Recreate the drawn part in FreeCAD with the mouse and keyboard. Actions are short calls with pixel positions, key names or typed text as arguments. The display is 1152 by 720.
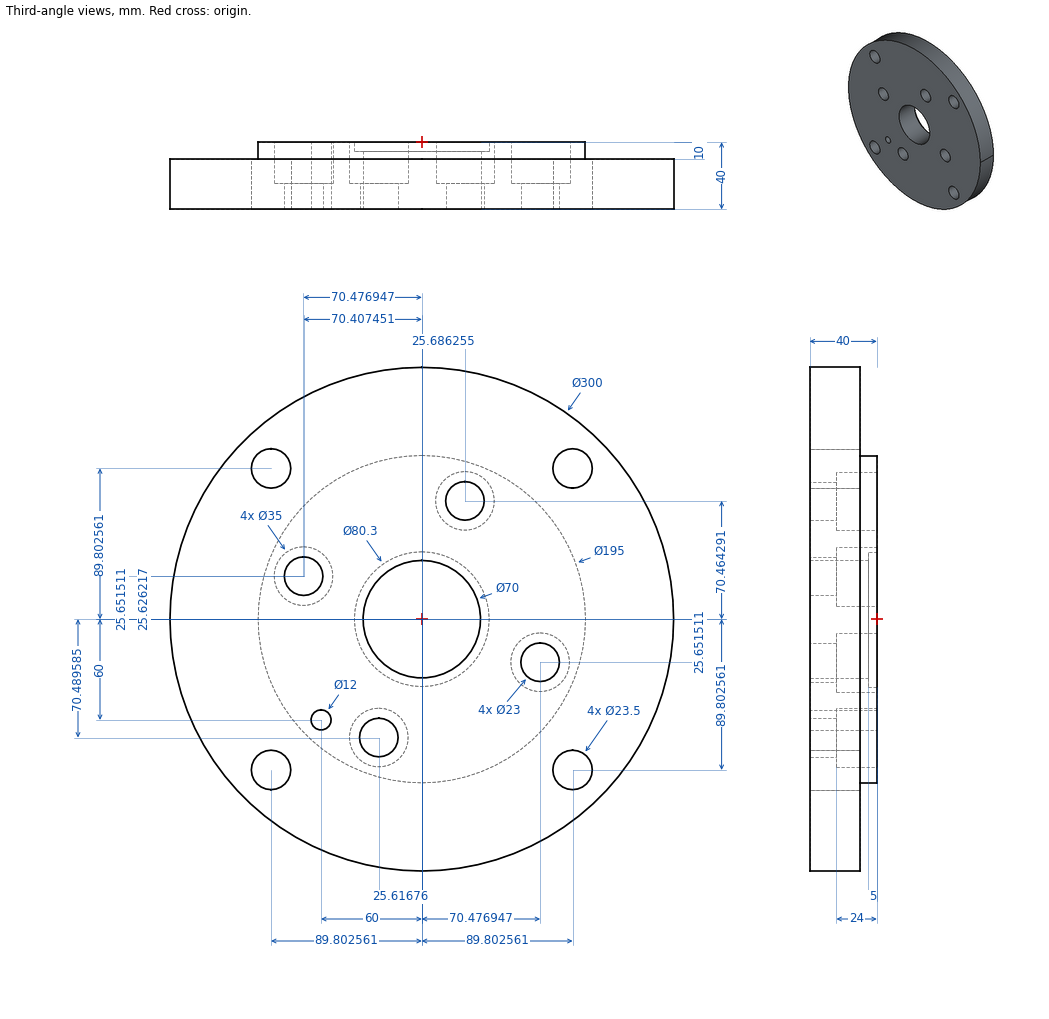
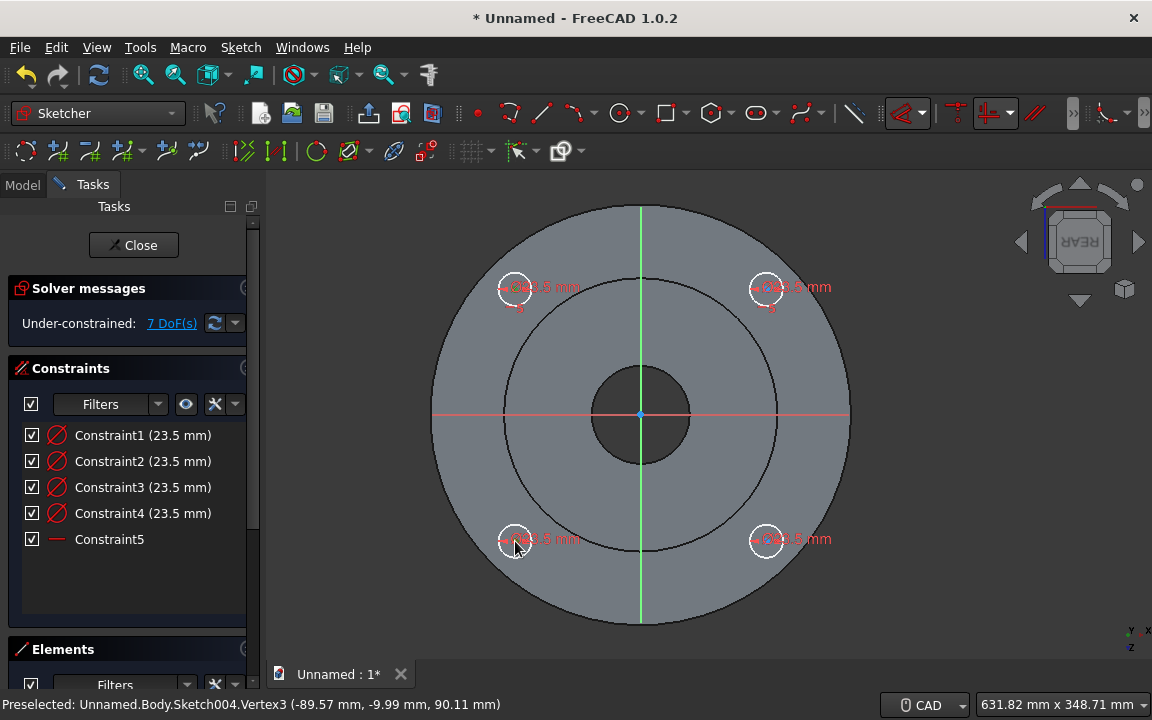
click(1012, 114)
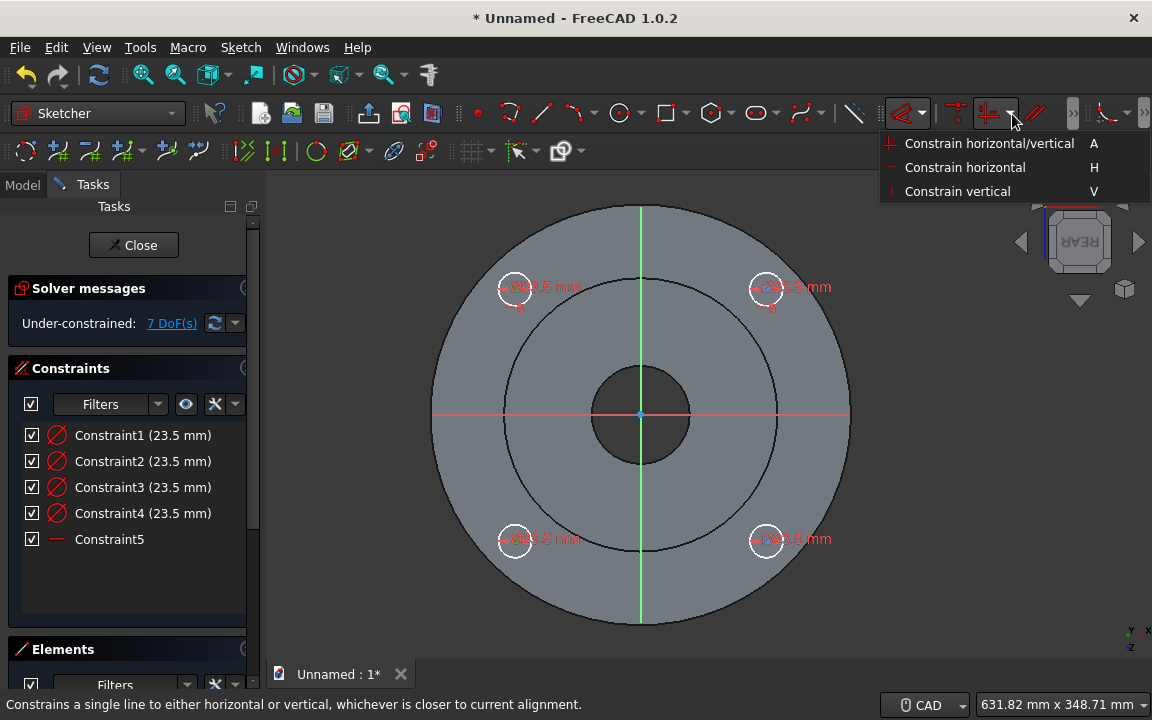
click(1015, 191)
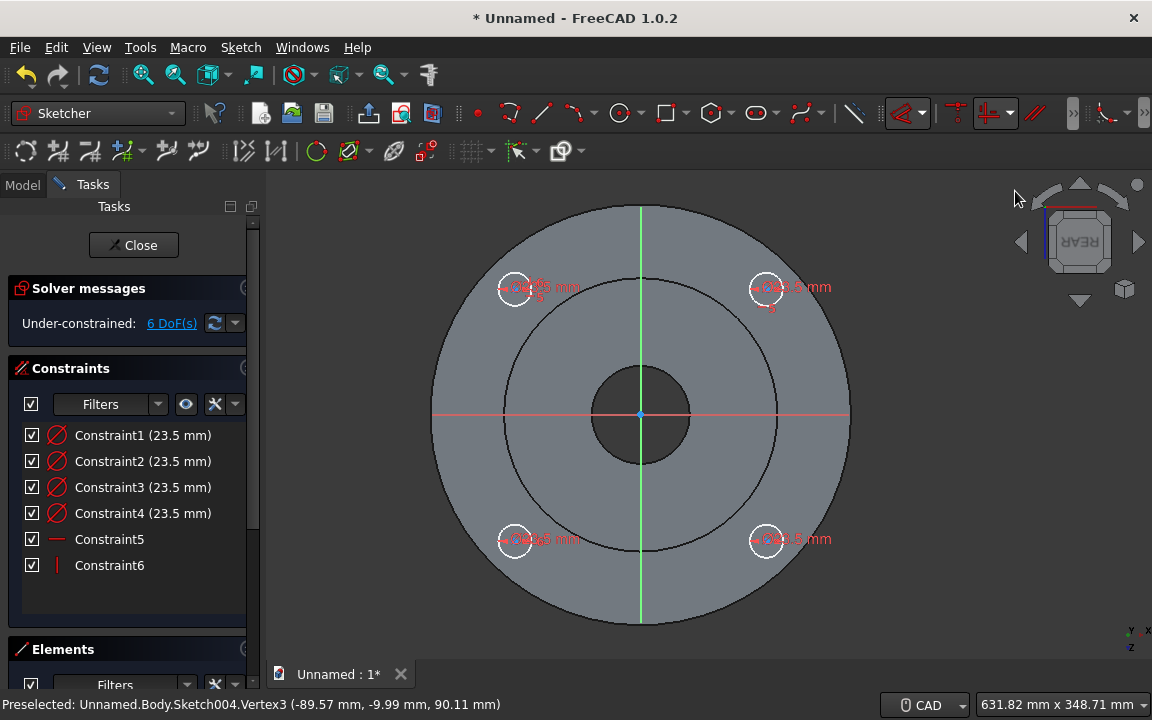
click(766, 289)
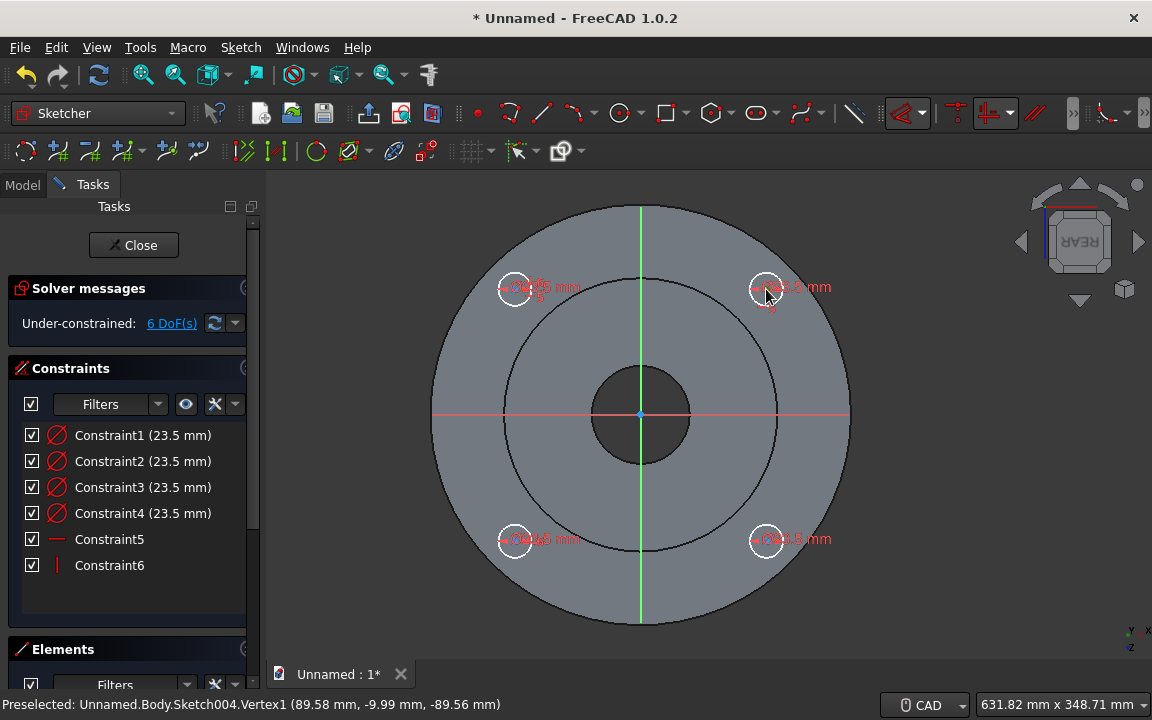
click(766, 541)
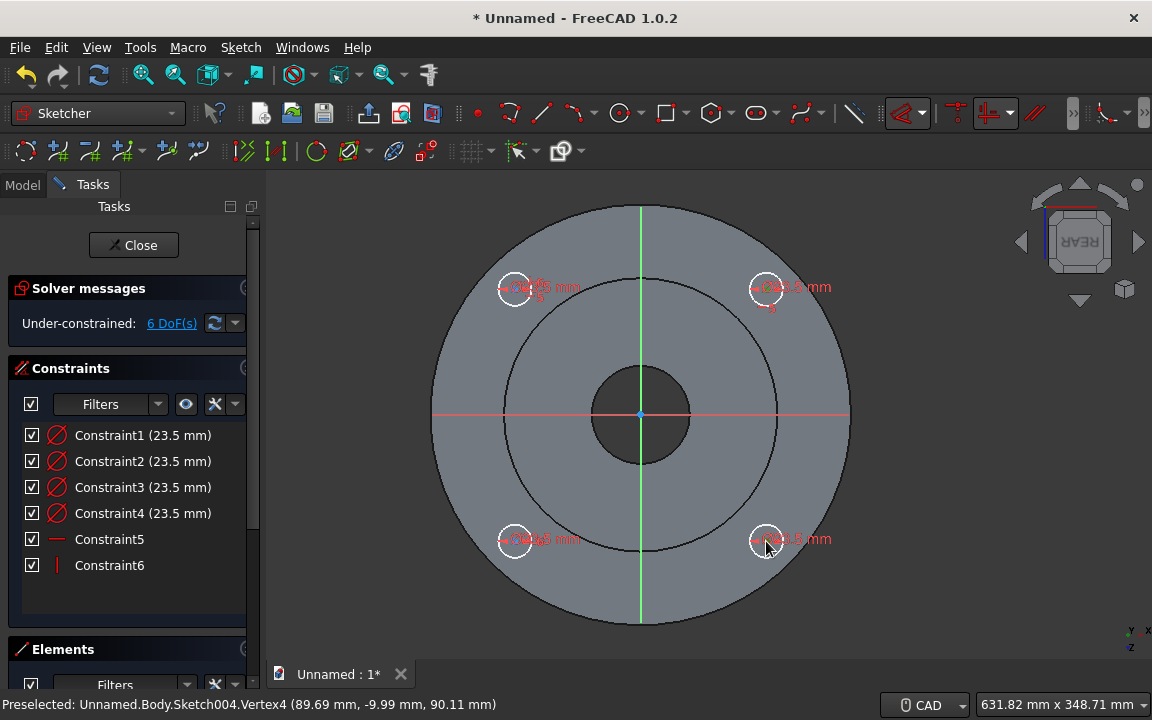
click(1012, 114)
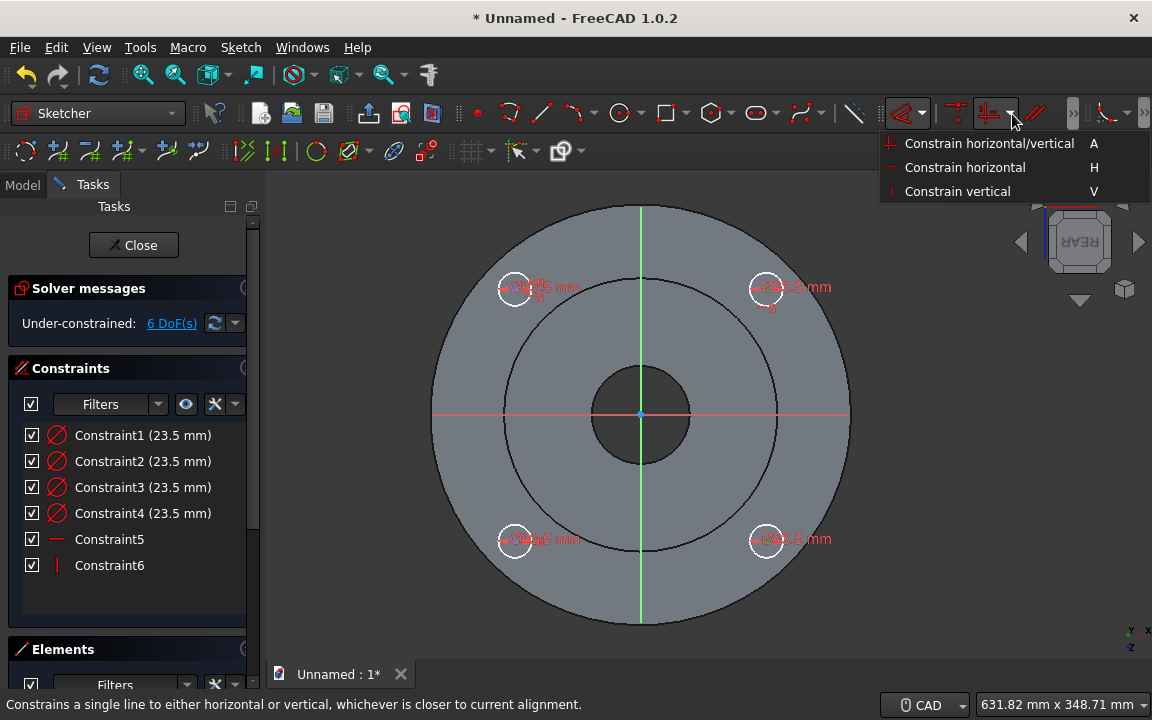
click(1015, 191)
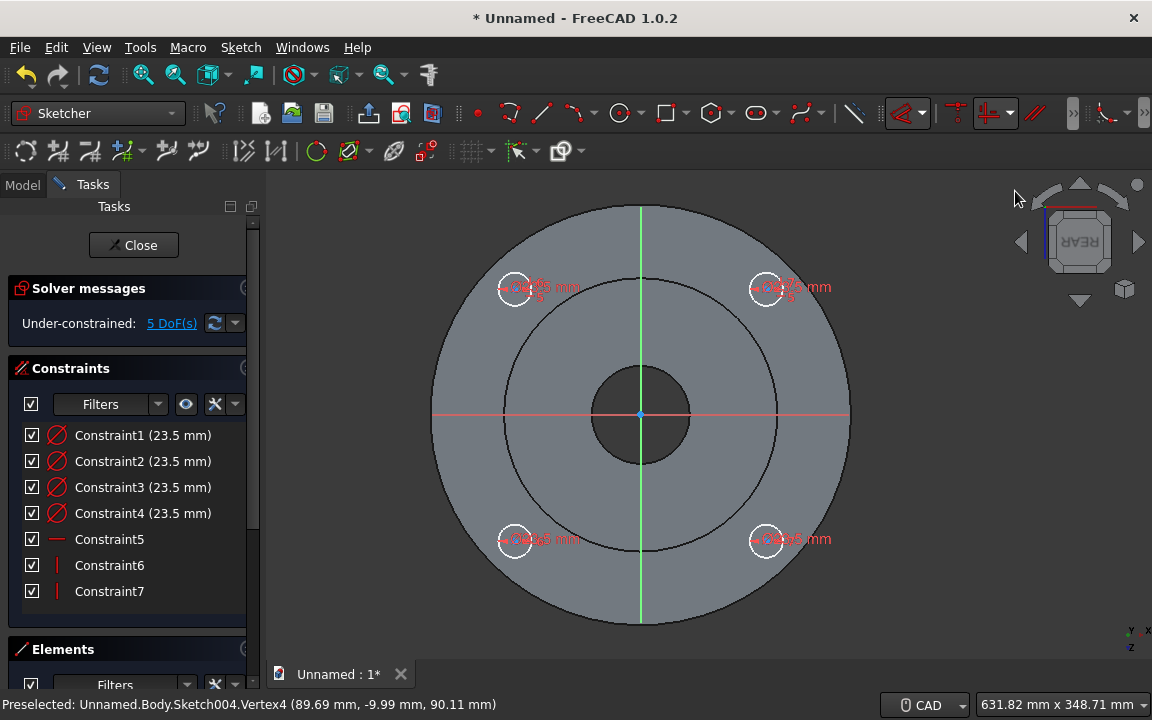
click(515, 541)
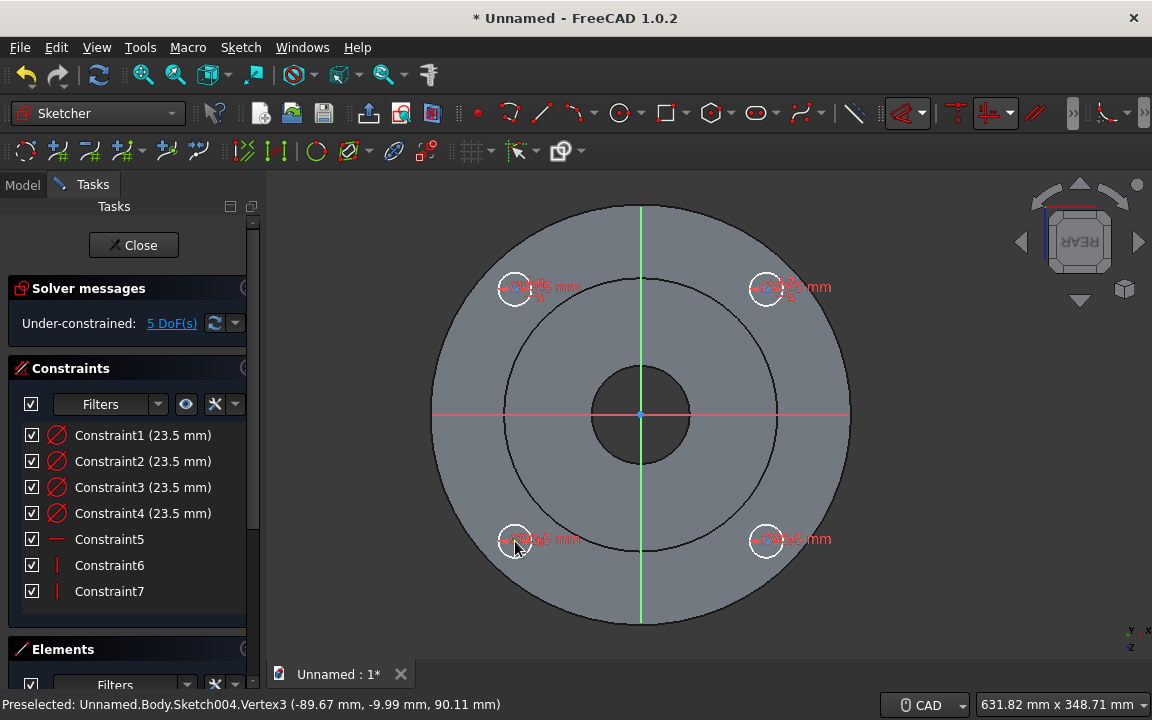
click(766, 541)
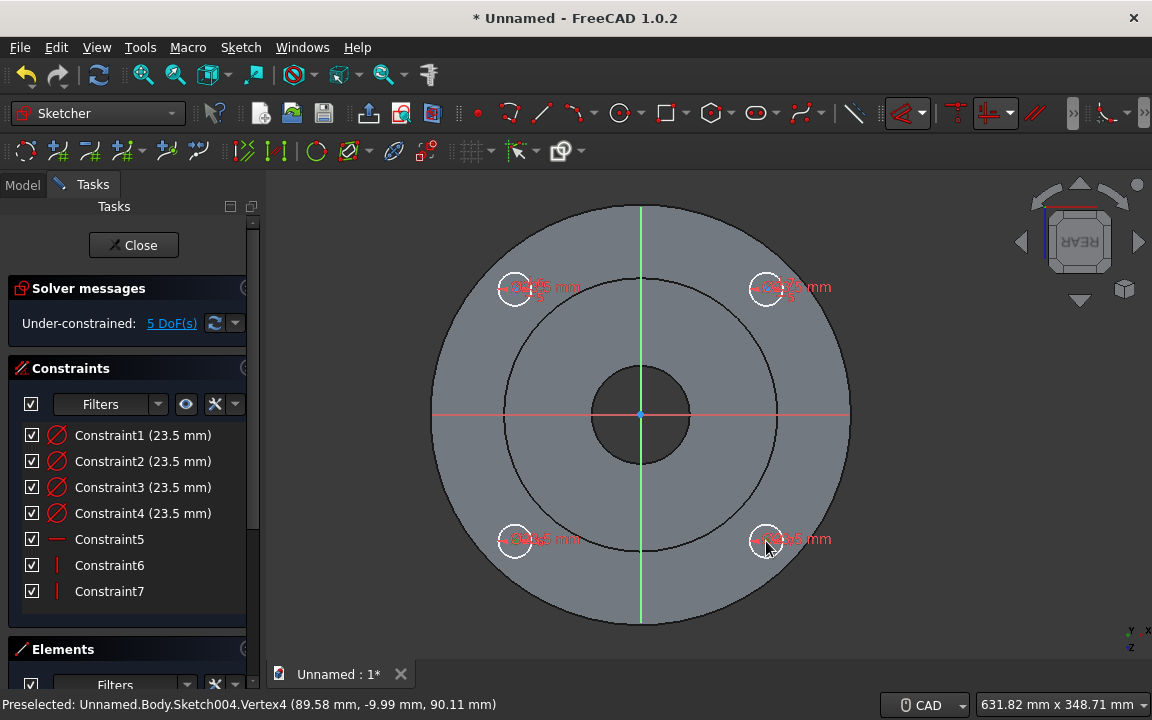
click(1012, 114)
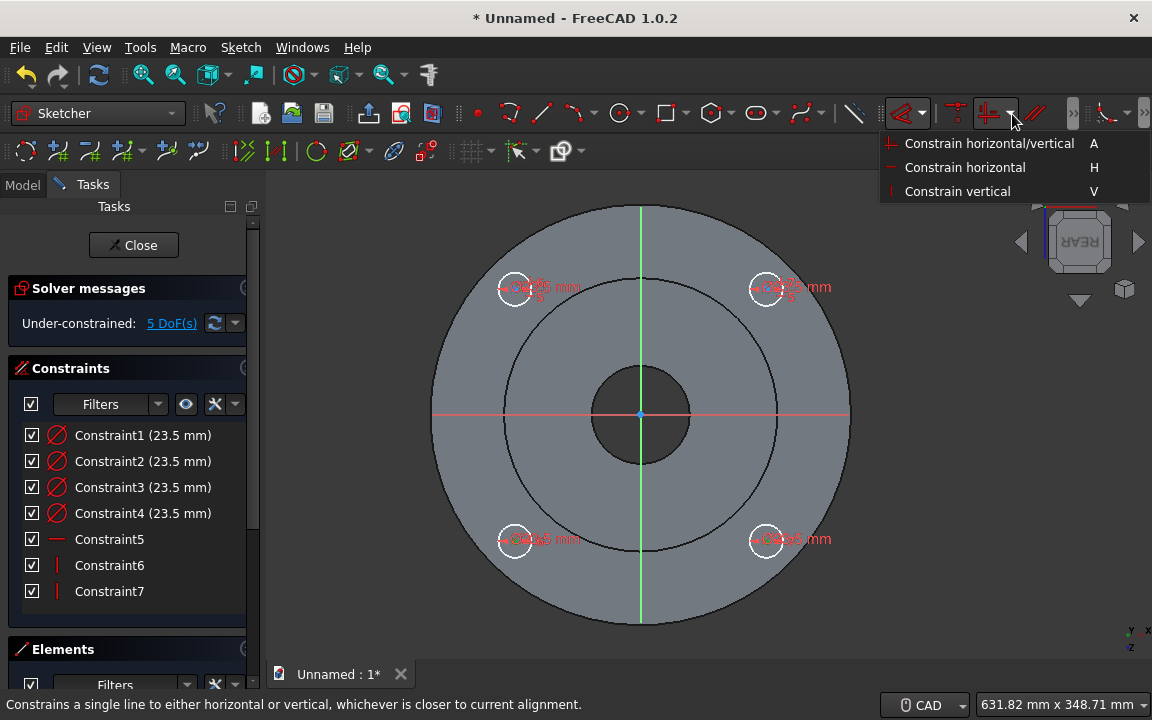
click(1015, 167)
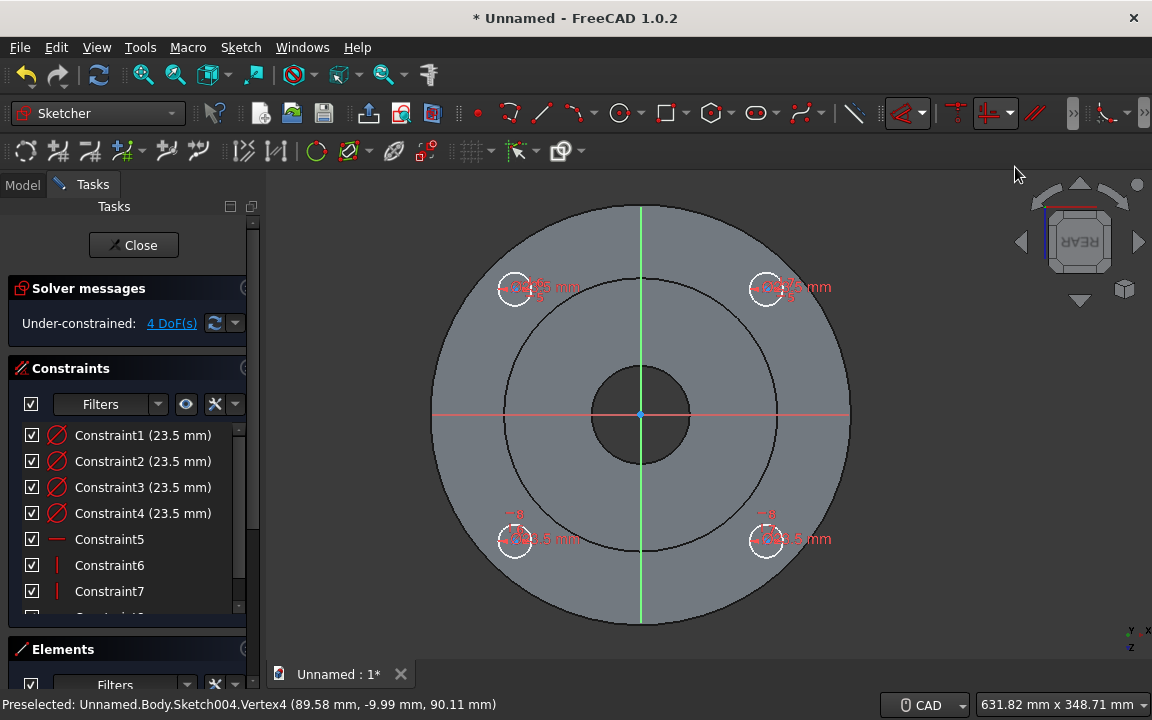
click(902, 114)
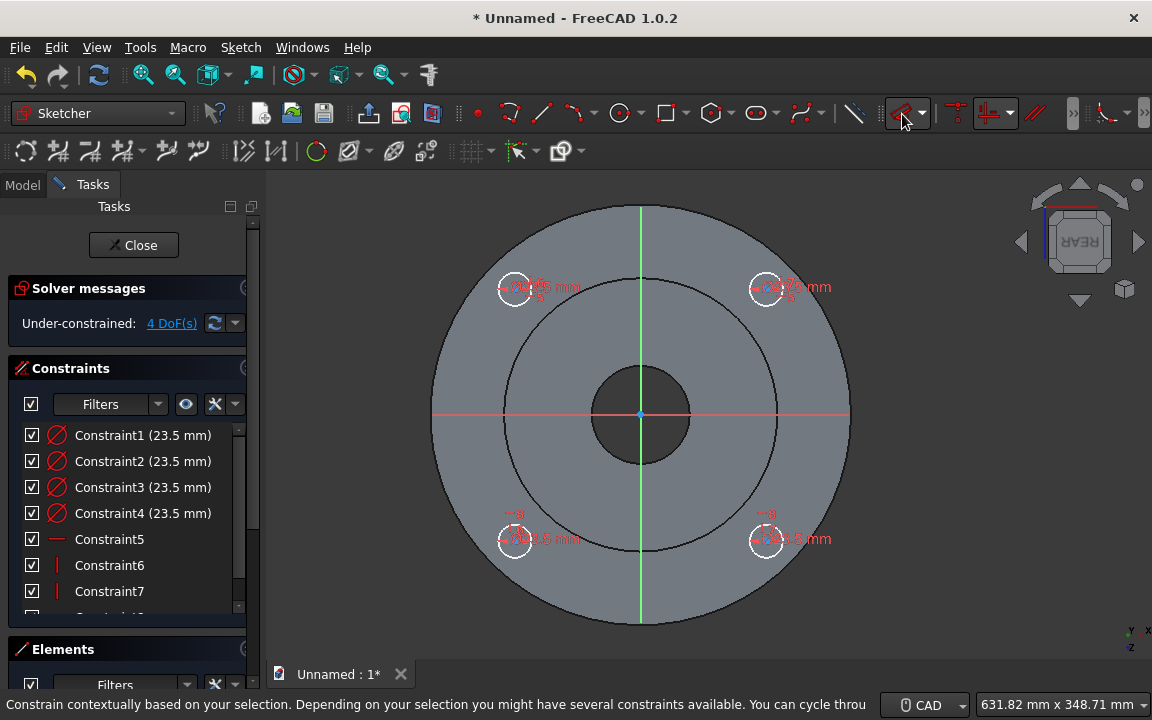
click(766, 289)
click(704, 255)